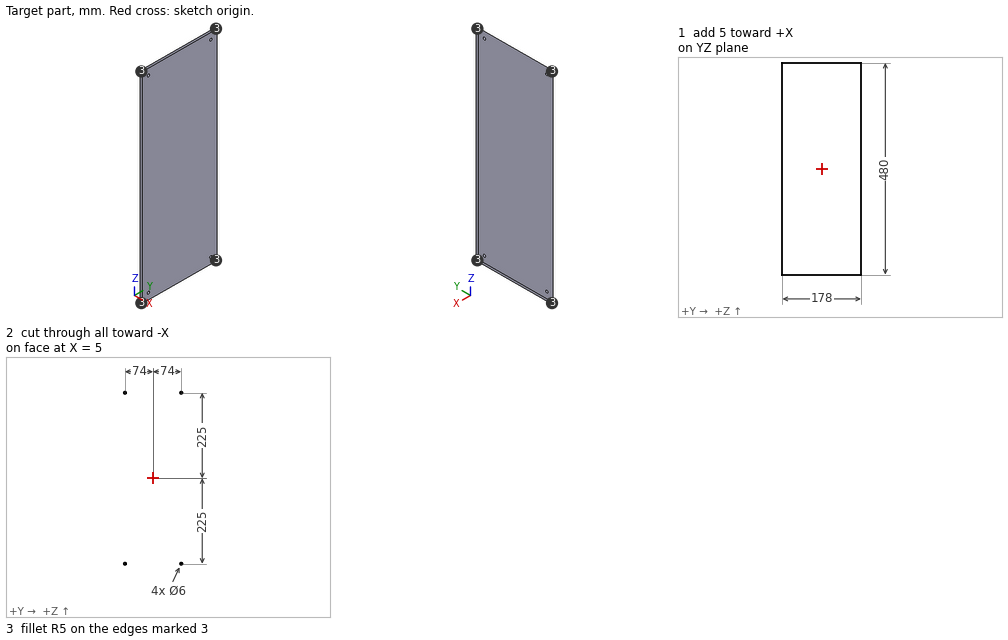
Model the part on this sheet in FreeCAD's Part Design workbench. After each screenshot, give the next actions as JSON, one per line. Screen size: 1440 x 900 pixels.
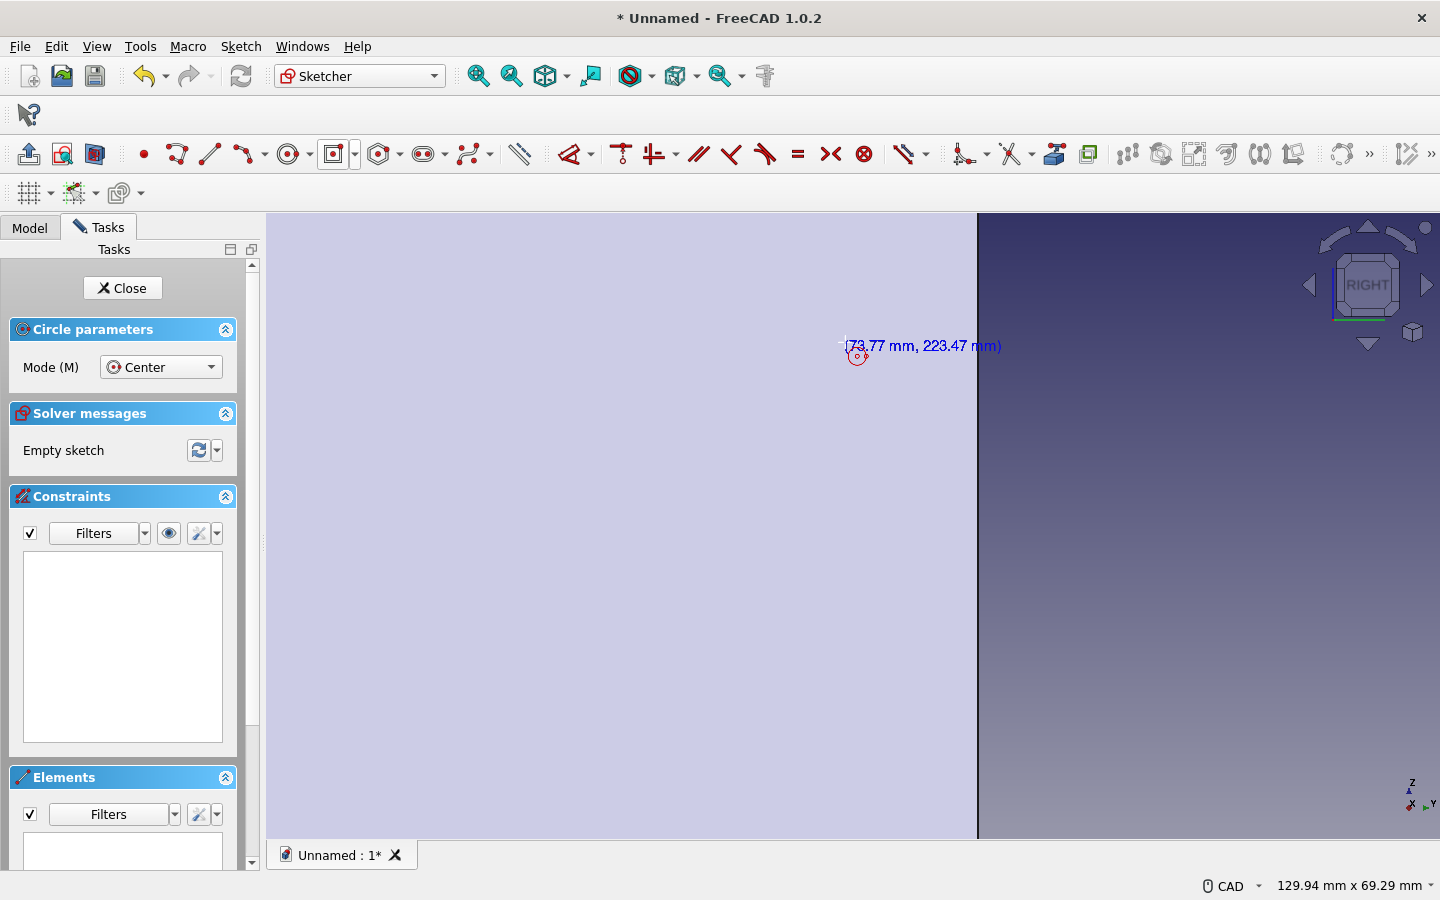
{"action": "scroll", "coordinate": [845, 342], "scroll_direction": "down", "scroll_amount": 12}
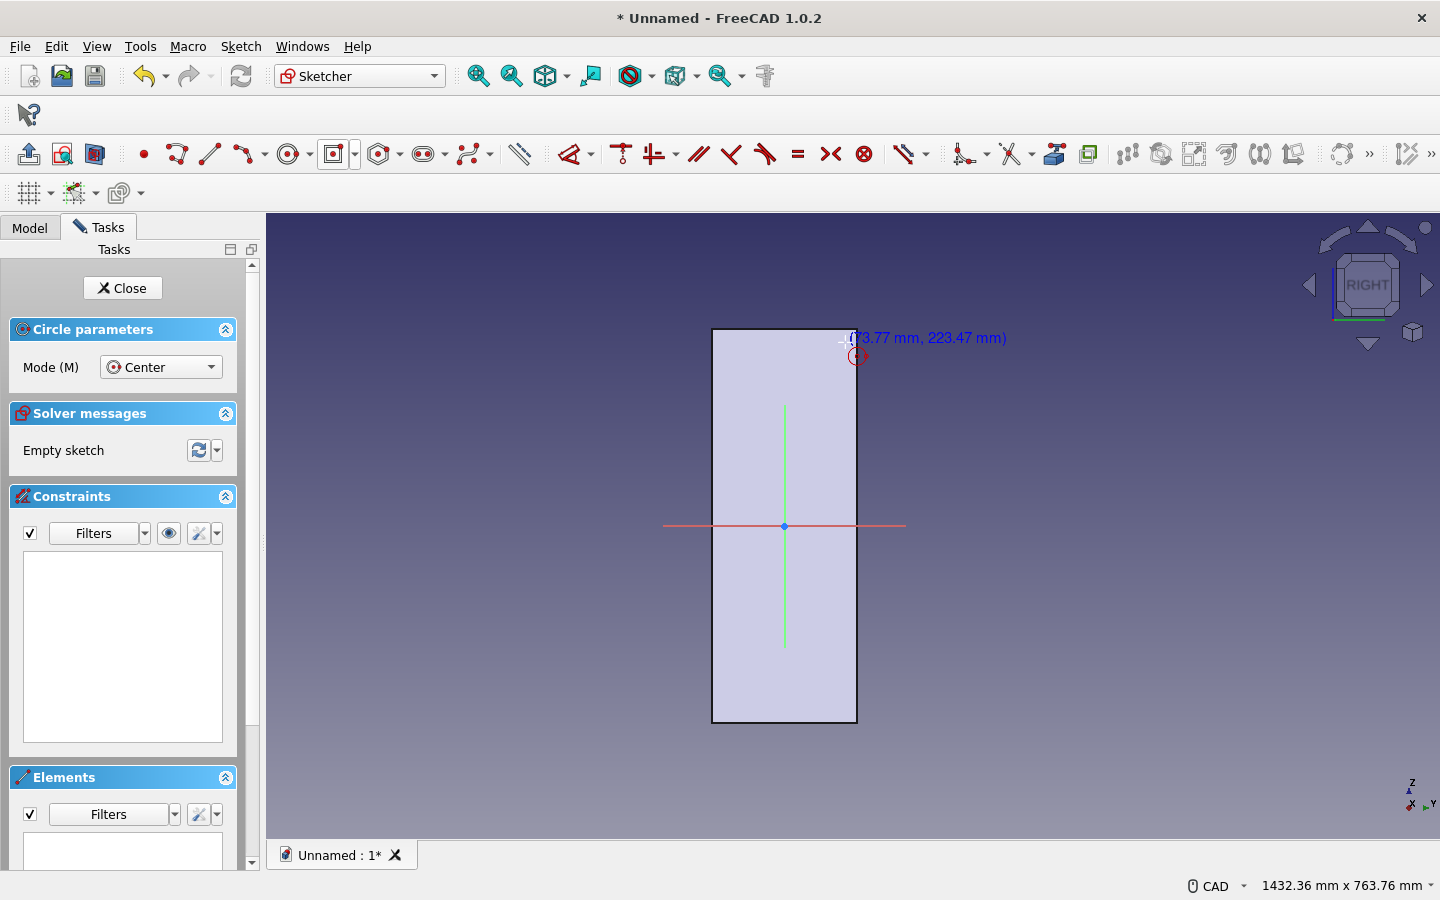
{"action": "left_click", "coordinate": [845, 342]}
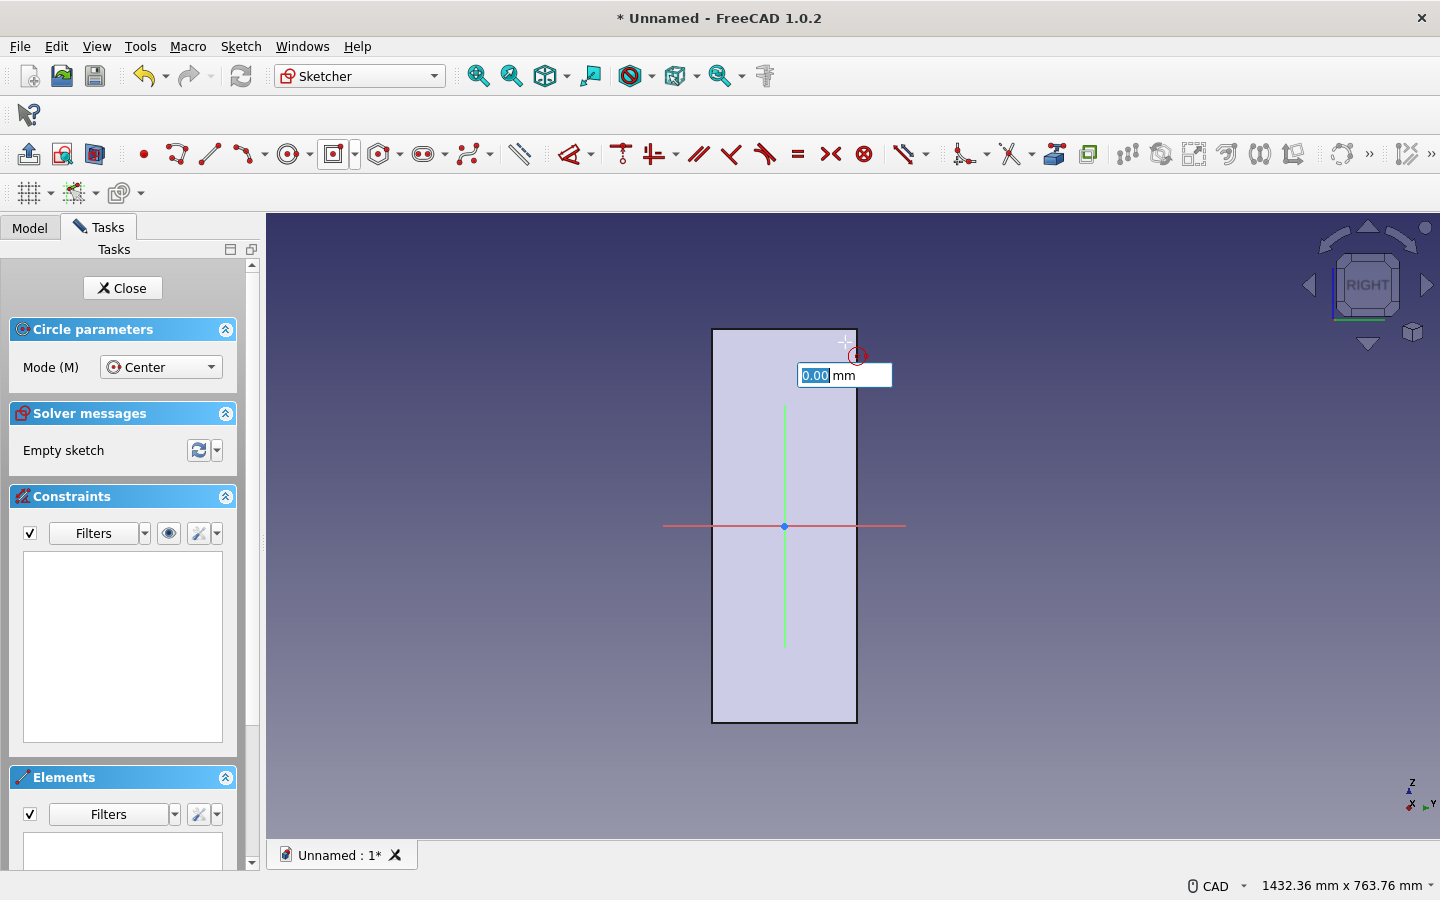
{"action": "scroll", "coordinate": [847, 340], "scroll_direction": "up", "scroll_amount": 10}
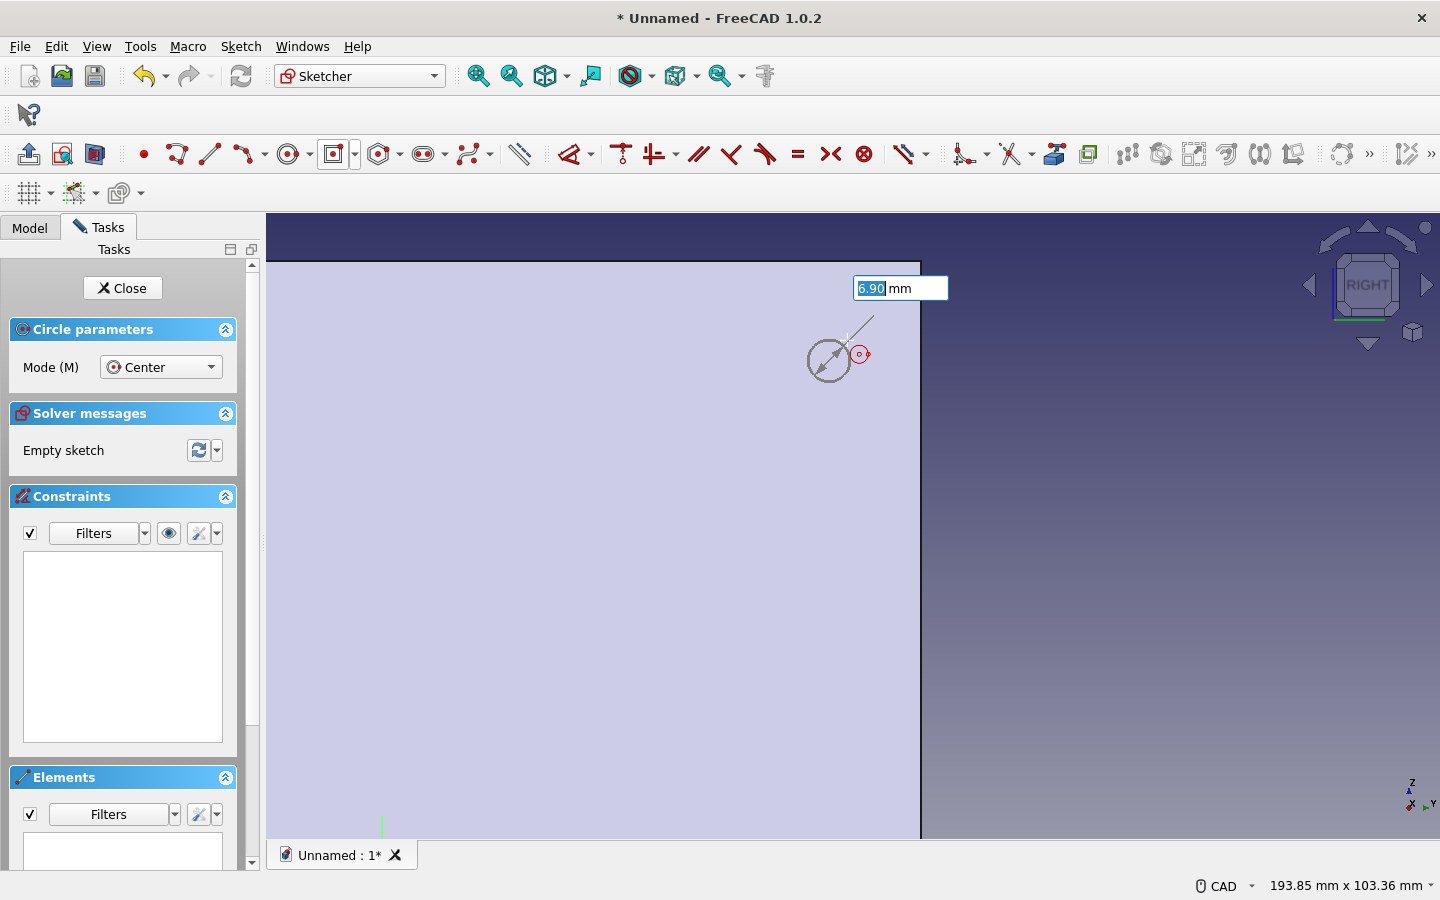
{"action": "left_click", "coordinate": [843, 339]}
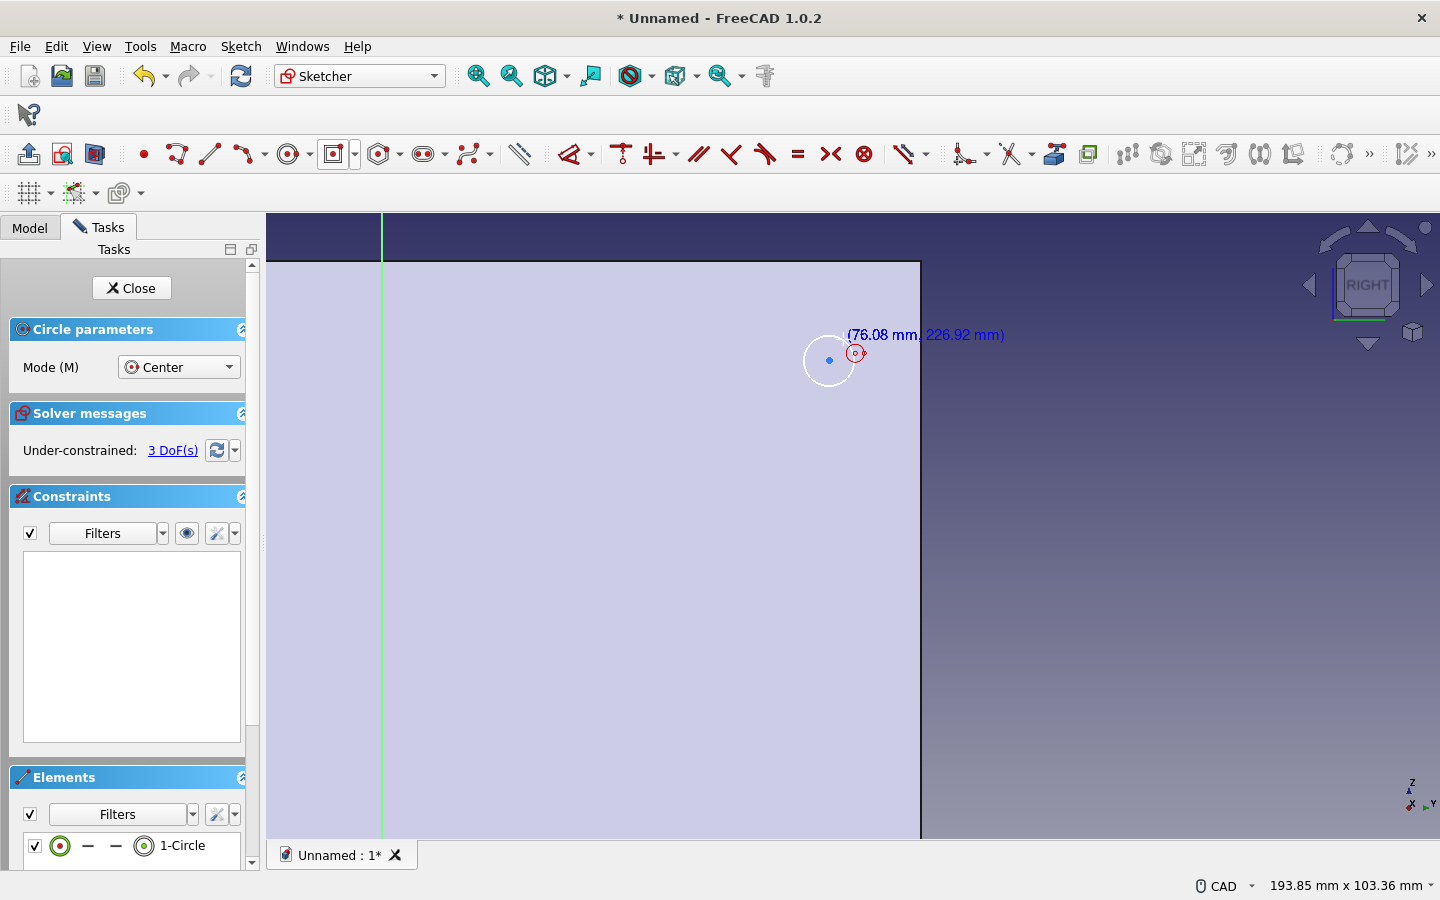
{"action": "scroll", "coordinate": [847, 340], "scroll_direction": "down", "scroll_amount": 10}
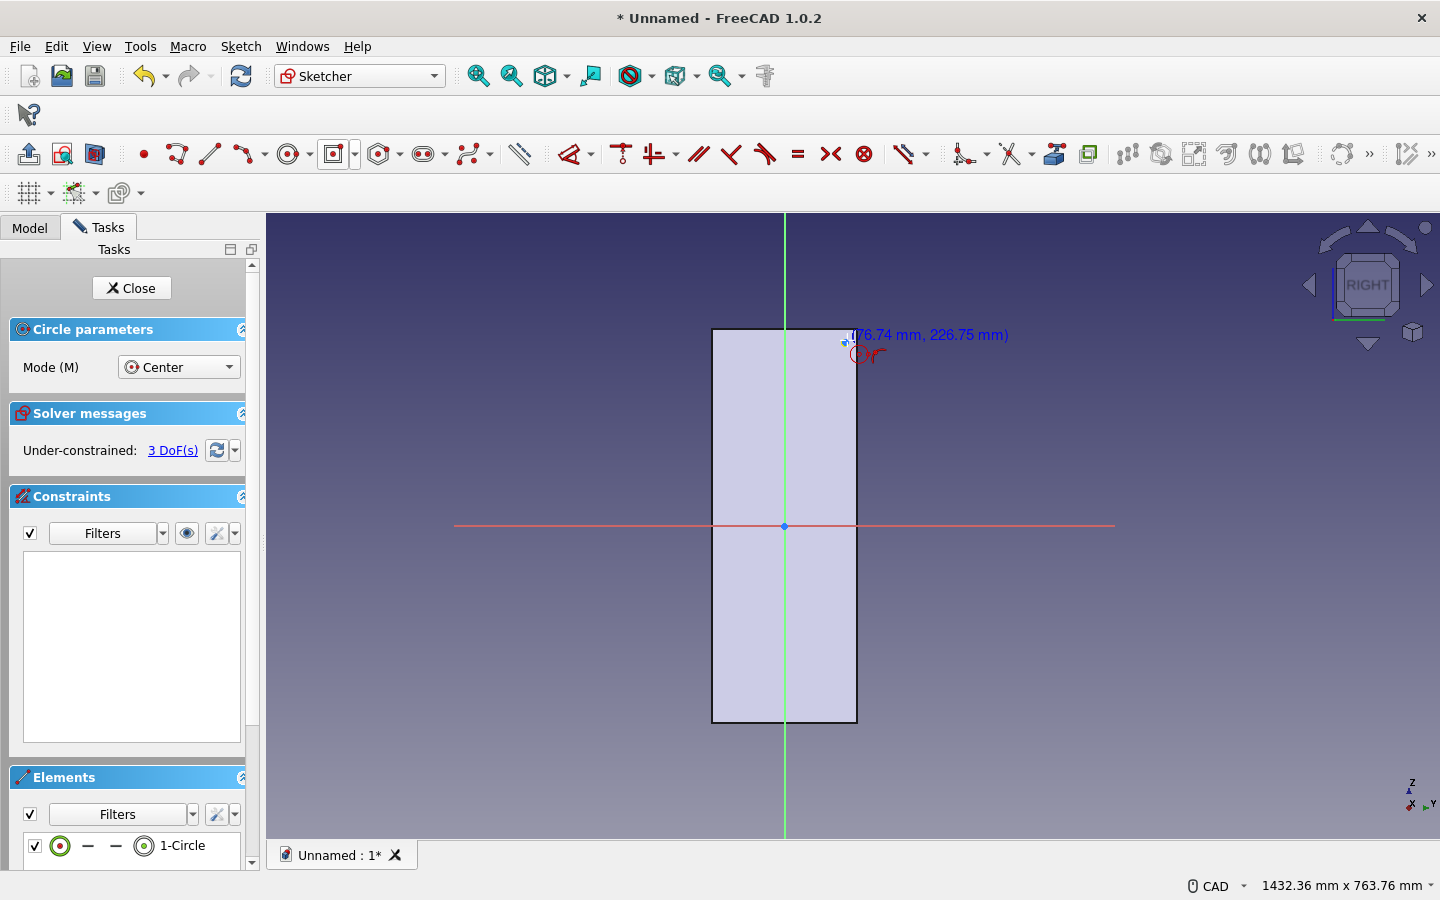
{"action": "scroll", "coordinate": [845, 711], "scroll_direction": "up", "scroll_amount": 12}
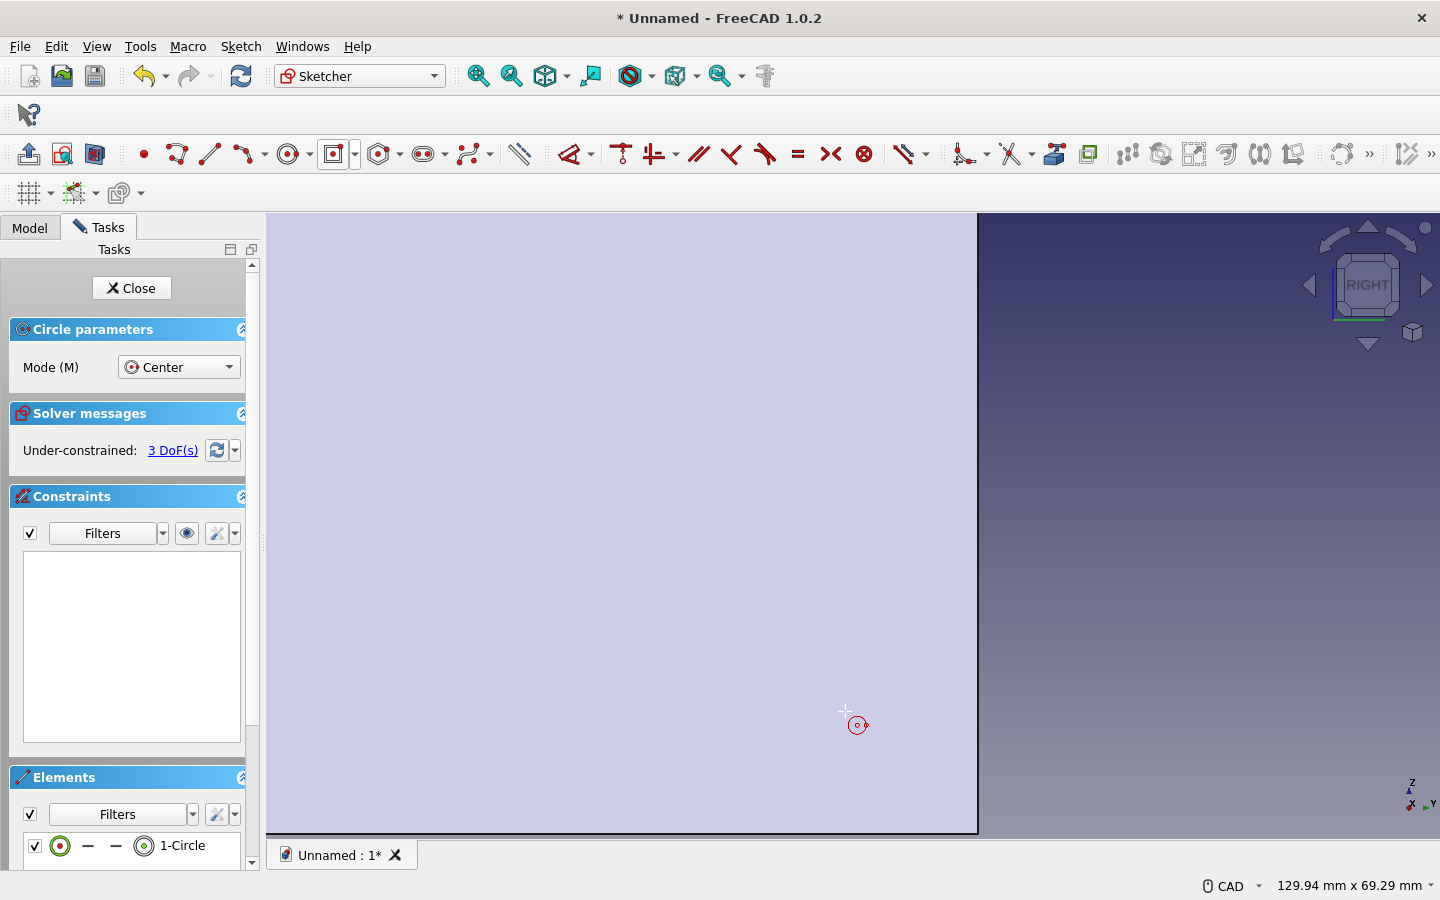
{"action": "scroll", "coordinate": [845, 712], "scroll_direction": "down", "scroll_amount": 12}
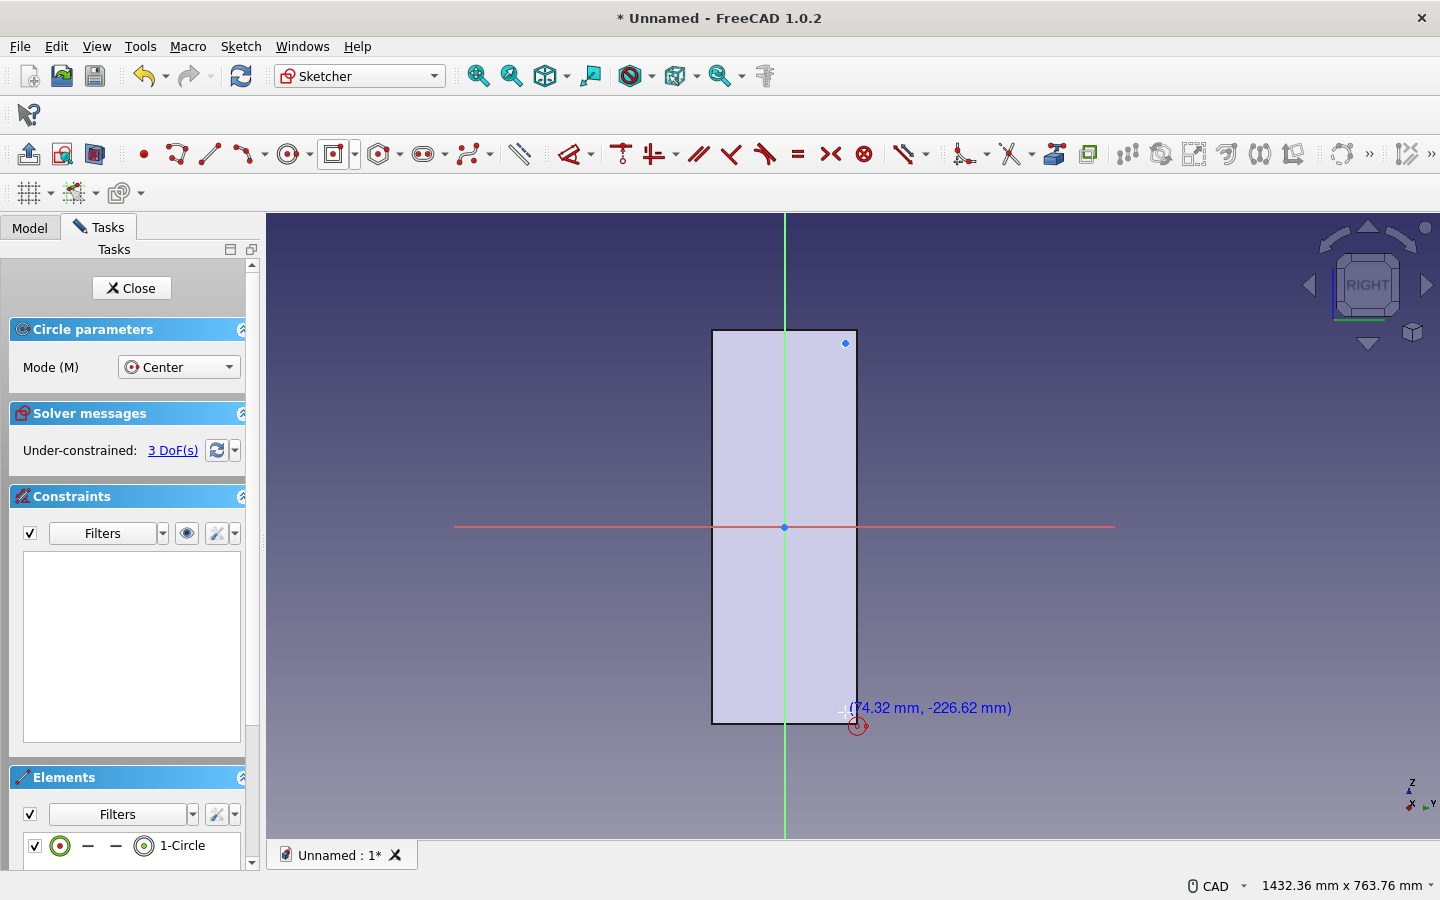
{"action": "left_click", "coordinate": [845, 711]}